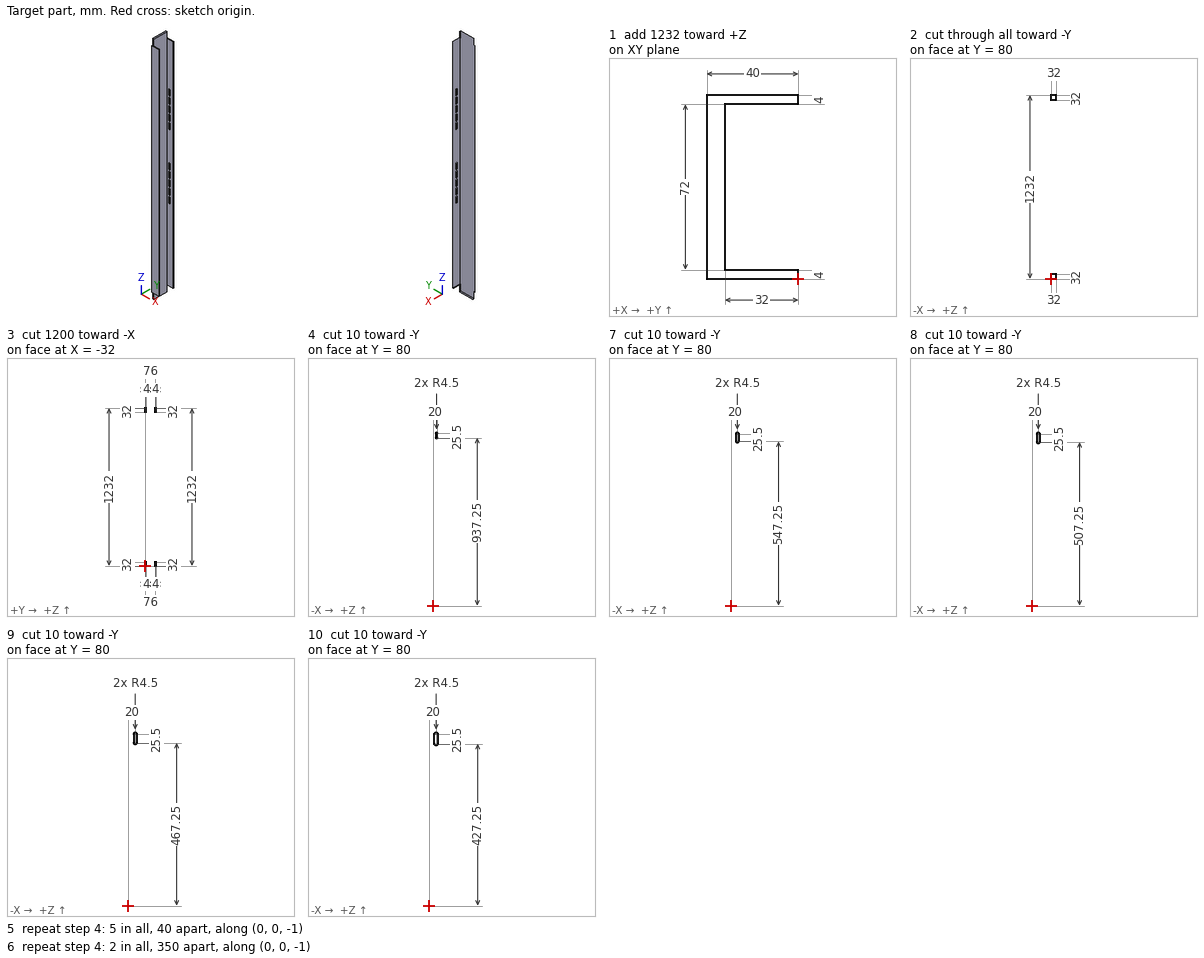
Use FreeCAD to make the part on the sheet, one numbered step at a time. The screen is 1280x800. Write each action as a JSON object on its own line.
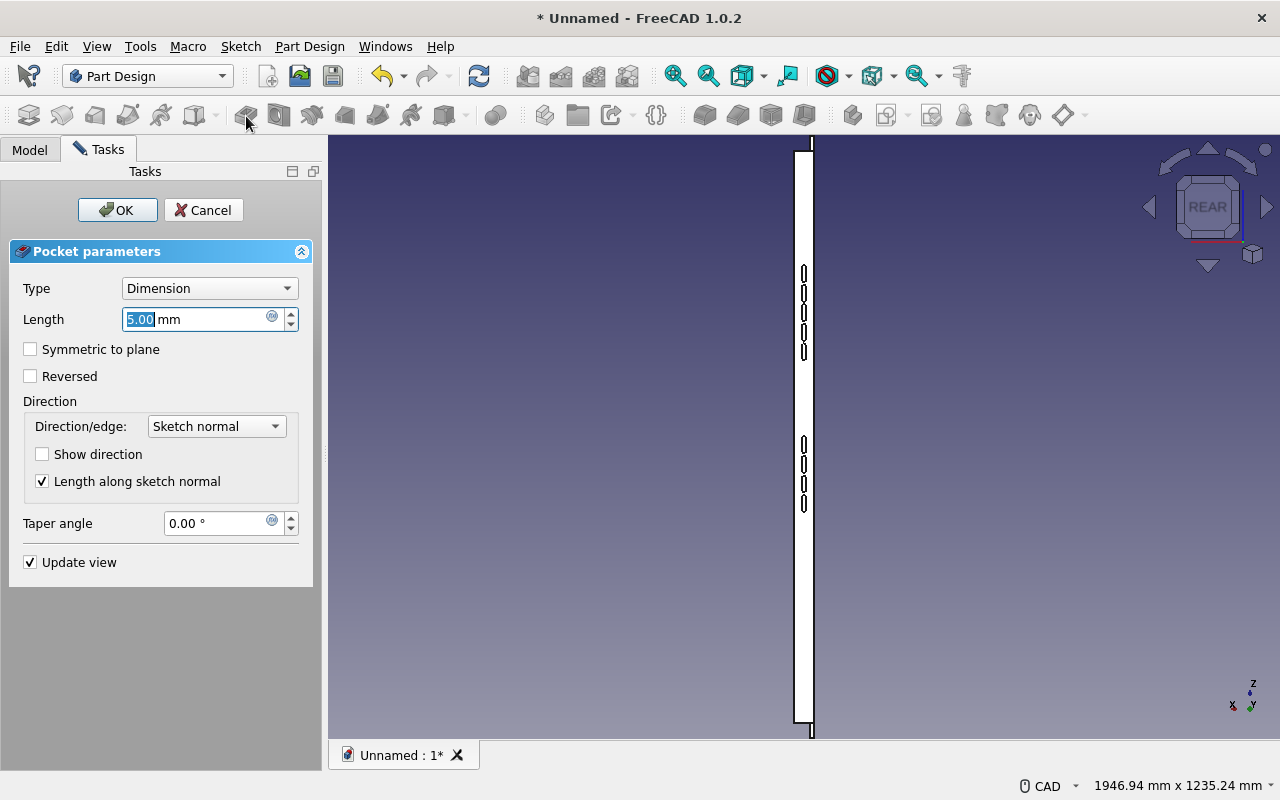
{"action": "type", "text": "10"}
{"action": "key", "text": "Tab"}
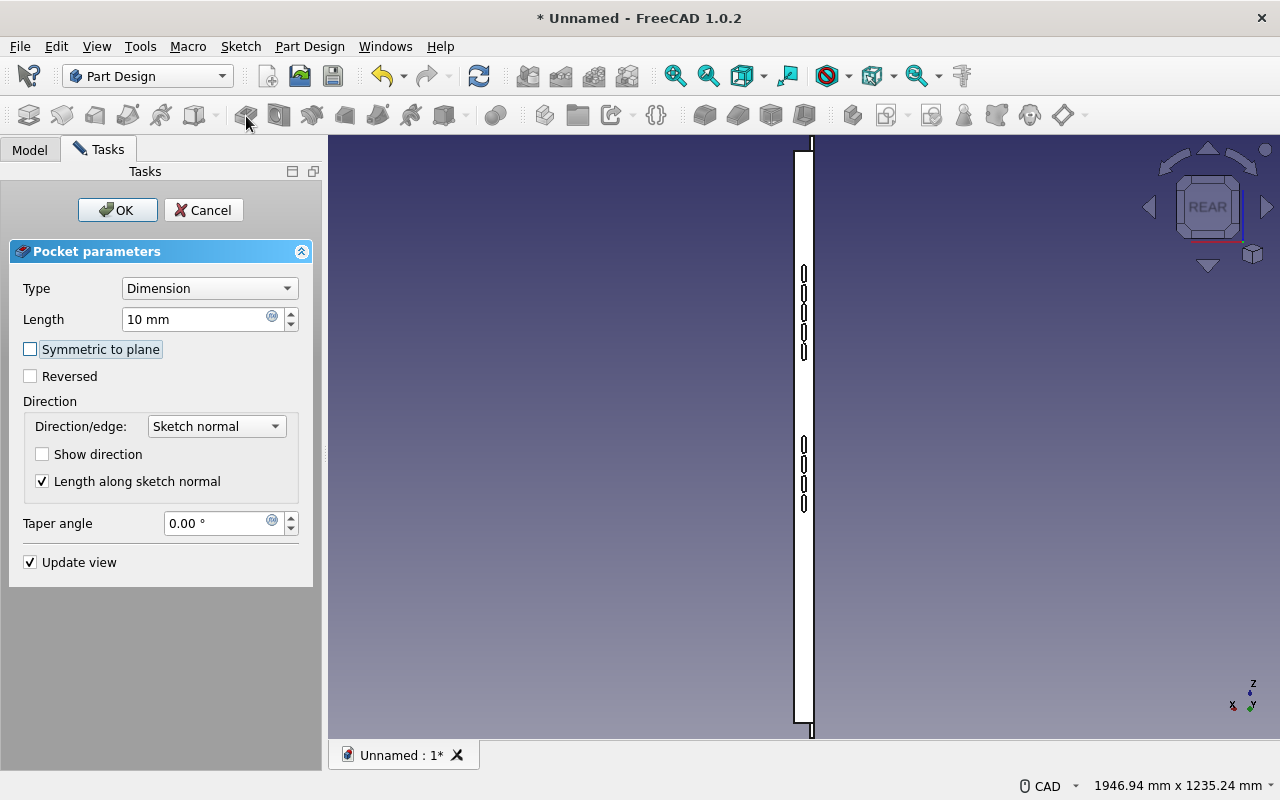
{"action": "left_click", "coordinate": [118, 210]}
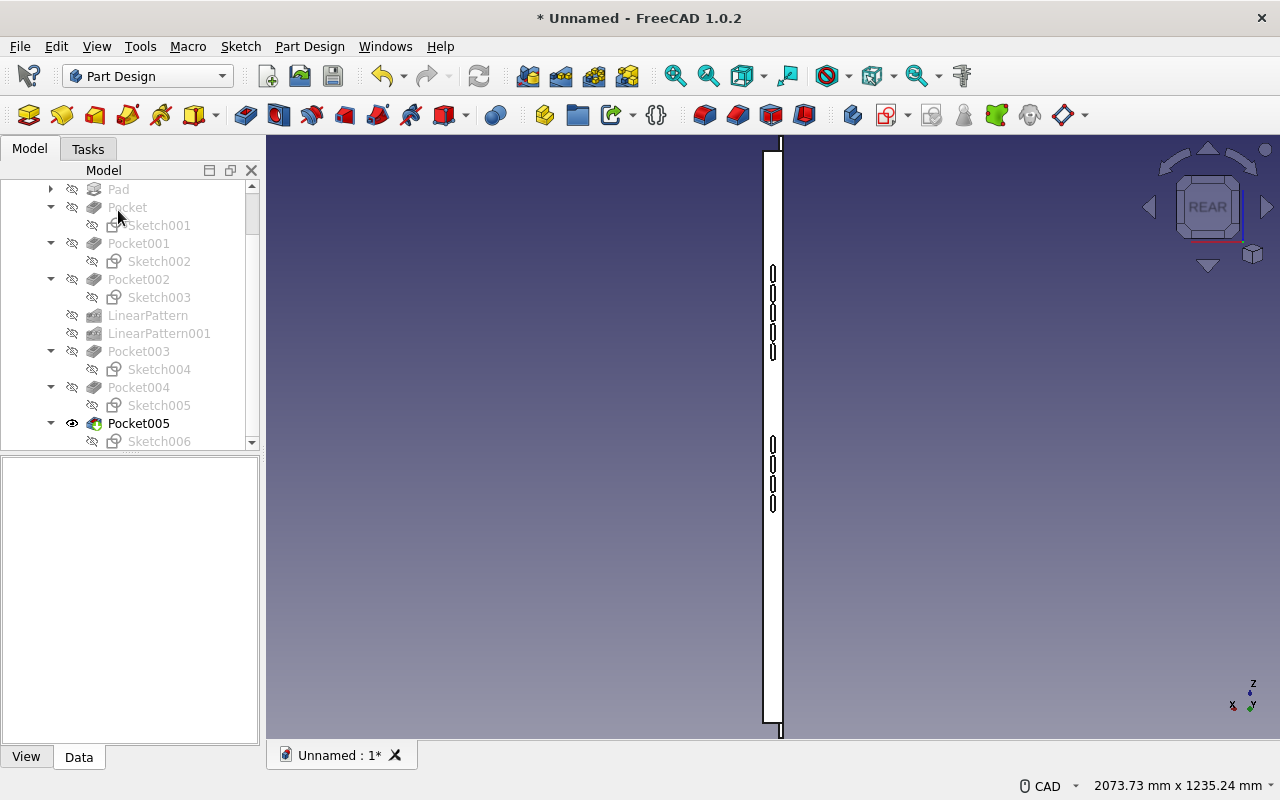
{"action": "left_click", "coordinate": [773, 191]}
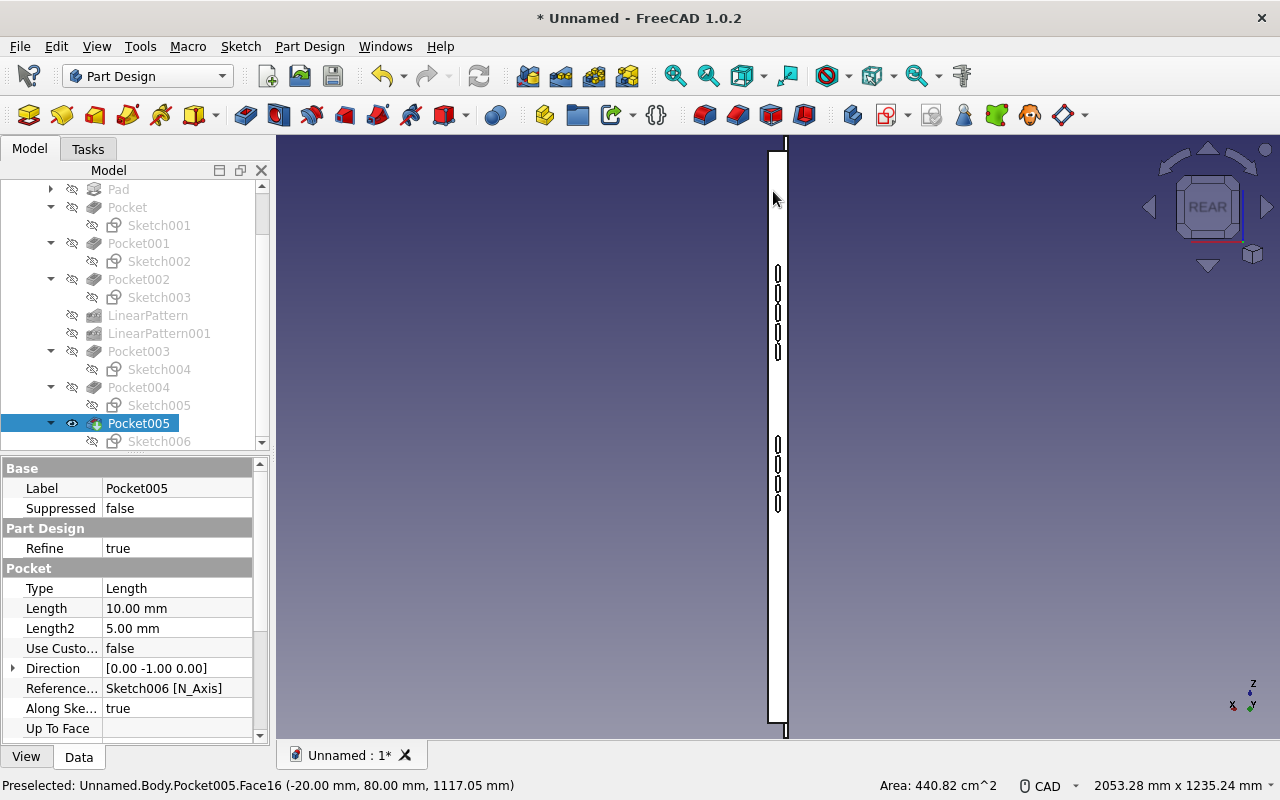
{"action": "left_click", "coordinate": [886, 116]}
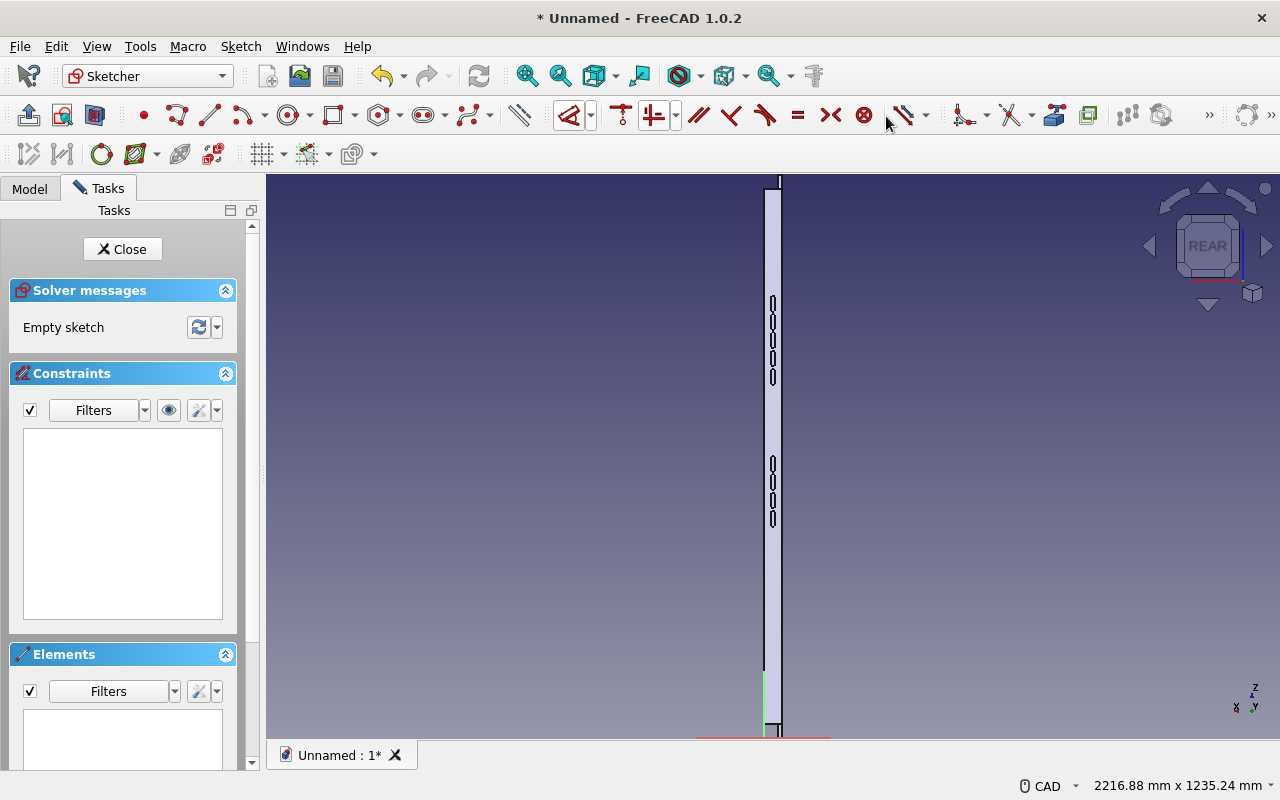
{"action": "scroll", "coordinate": [777, 541], "scroll_direction": "up", "scroll_amount": 15}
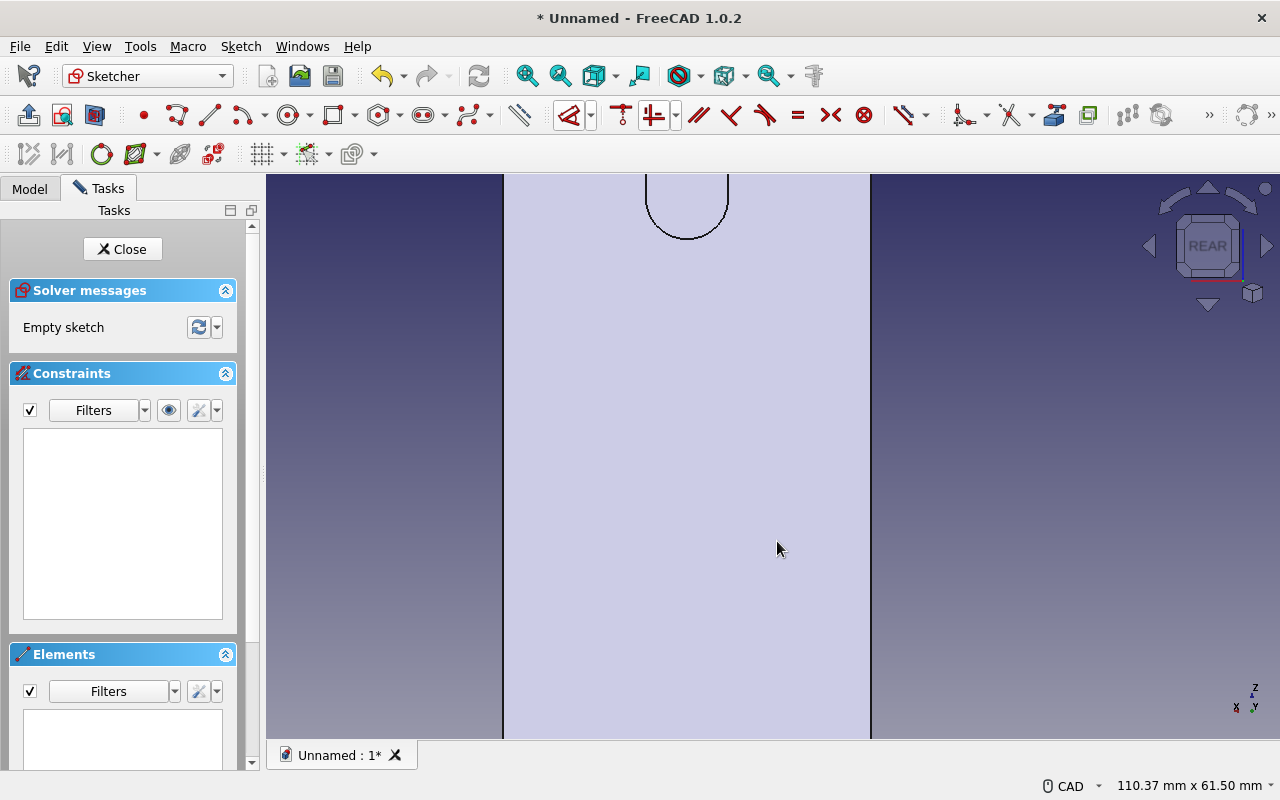
{"action": "left_click", "coordinate": [422, 116]}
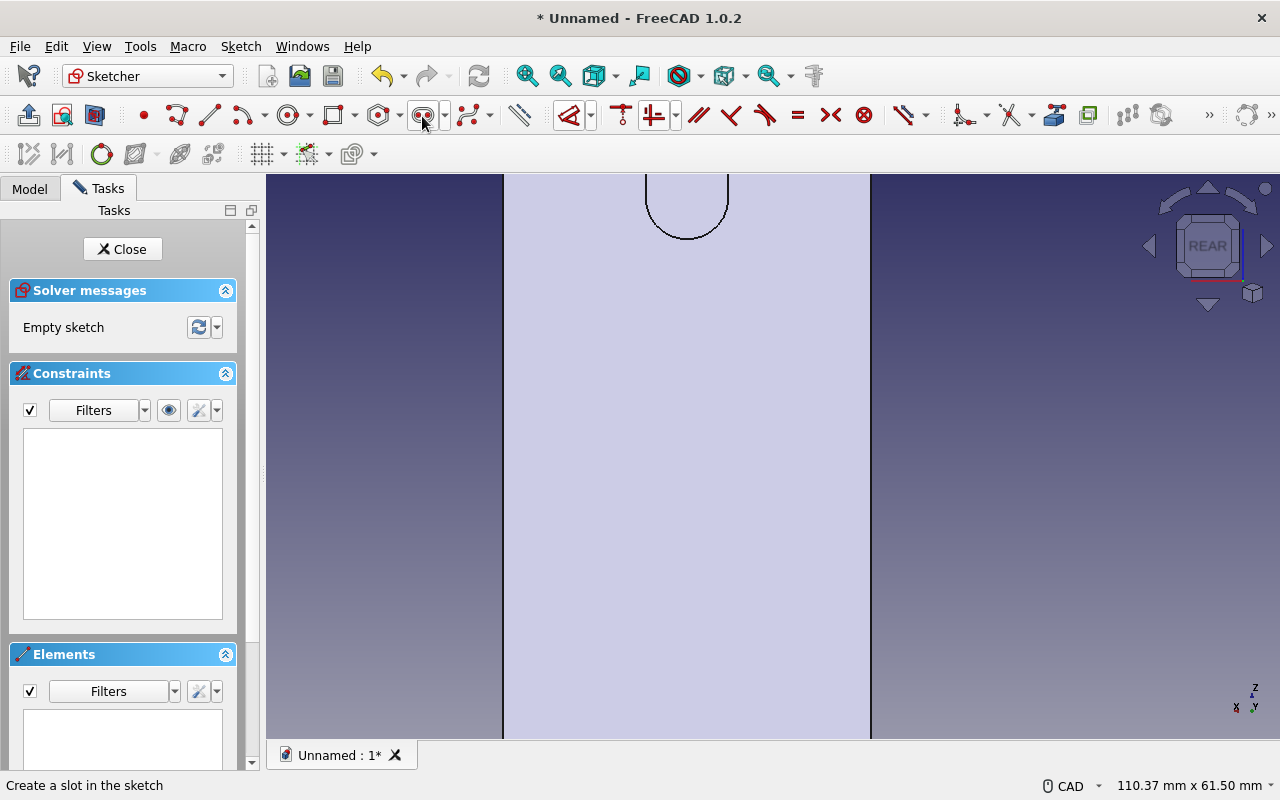
{"action": "left_click", "coordinate": [687, 565]}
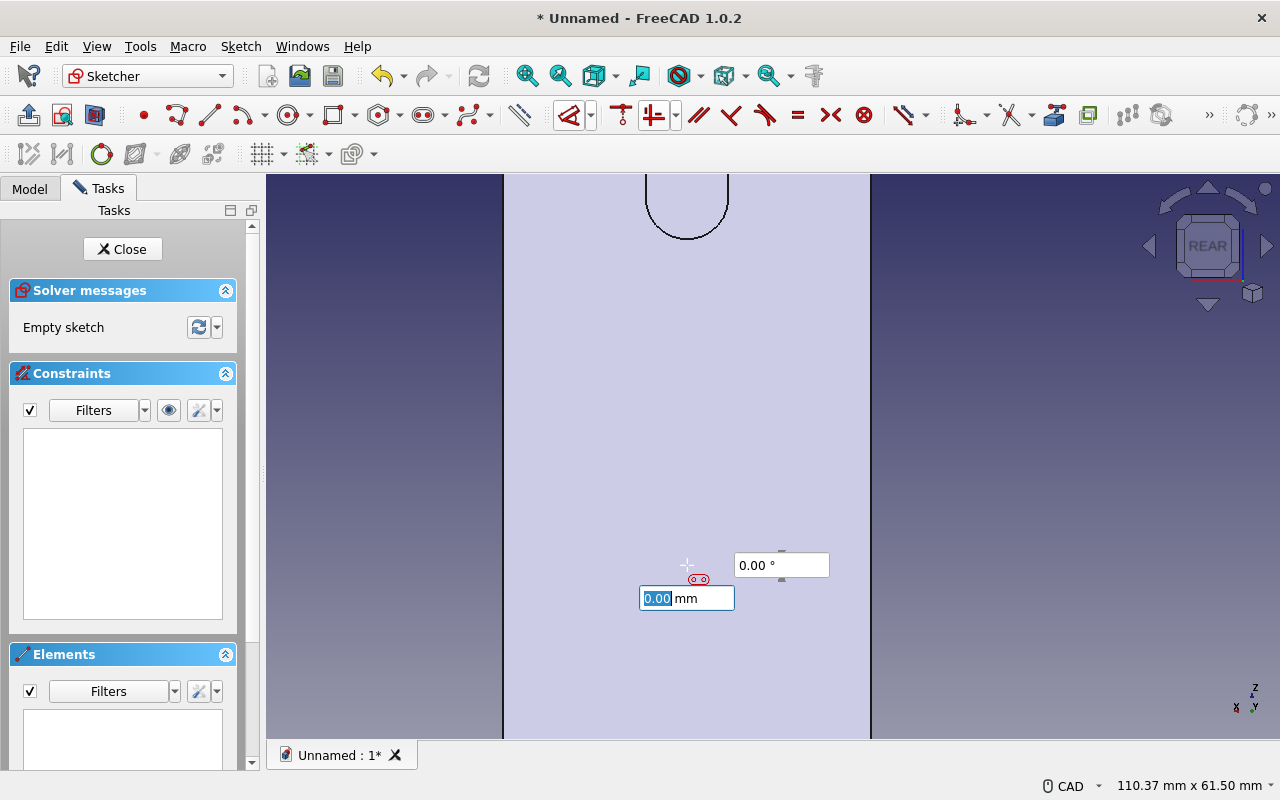
{"action": "left_click", "coordinate": [687, 331]}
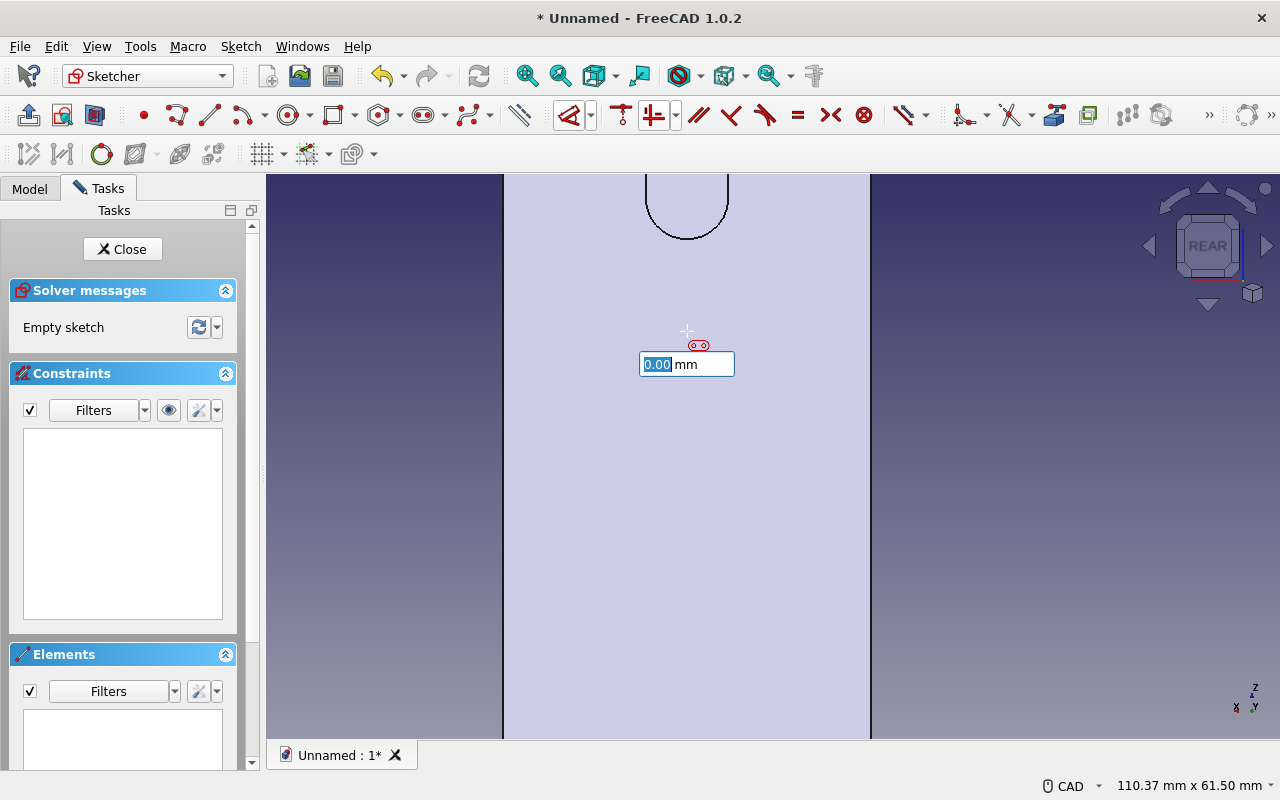
{"action": "left_click", "coordinate": [728, 448]}
{"action": "key", "text": "Escape"}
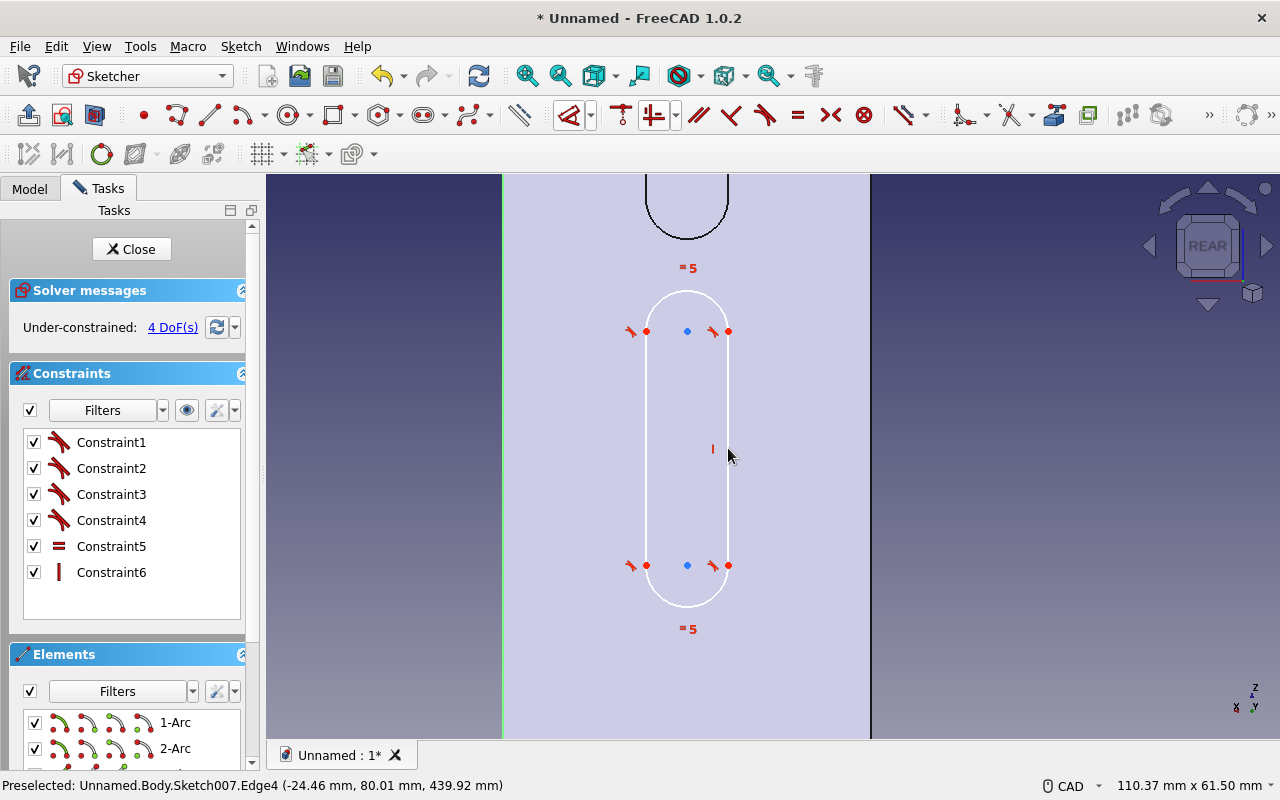
{"action": "left_click", "coordinate": [663, 599]}